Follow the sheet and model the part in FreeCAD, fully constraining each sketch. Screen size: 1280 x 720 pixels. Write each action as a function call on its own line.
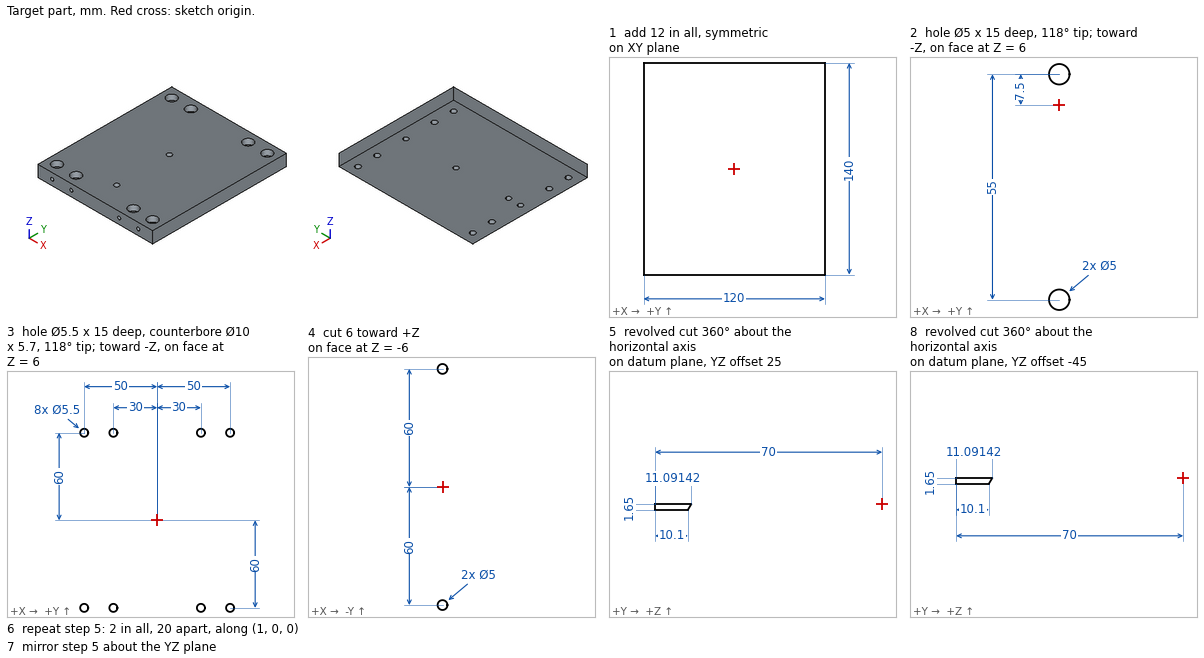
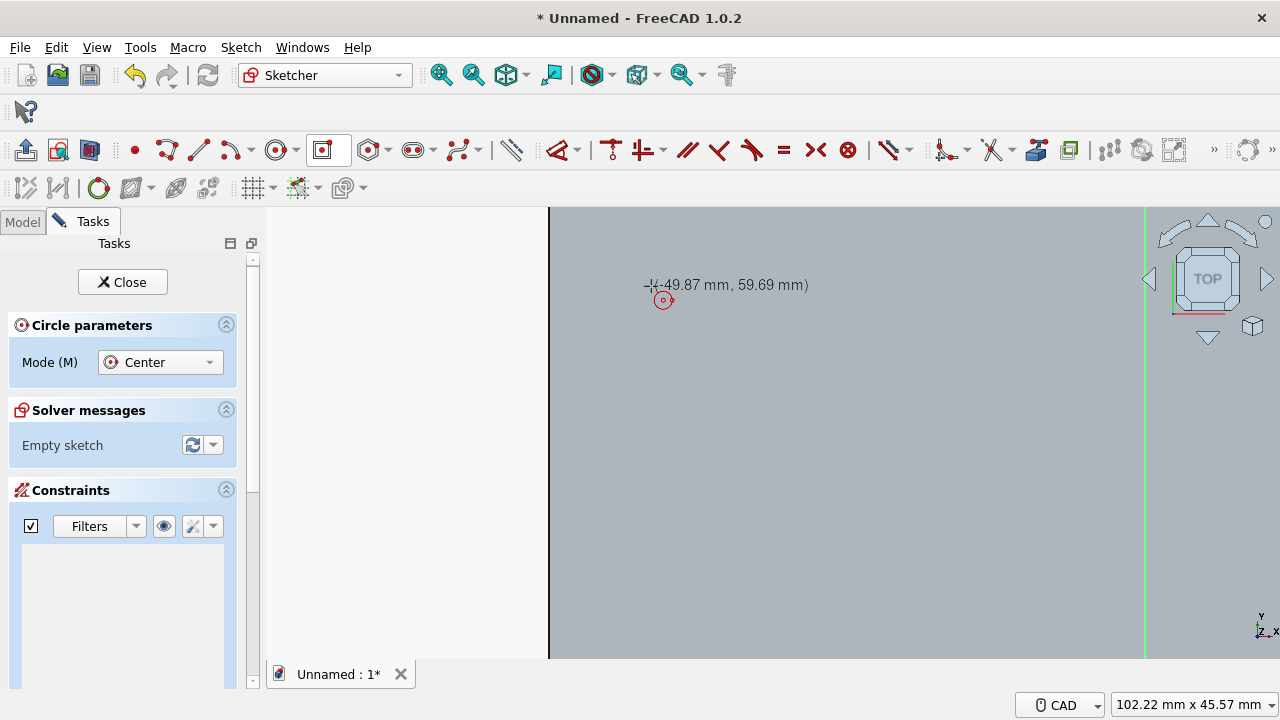
scroll(560, 286, down, 7)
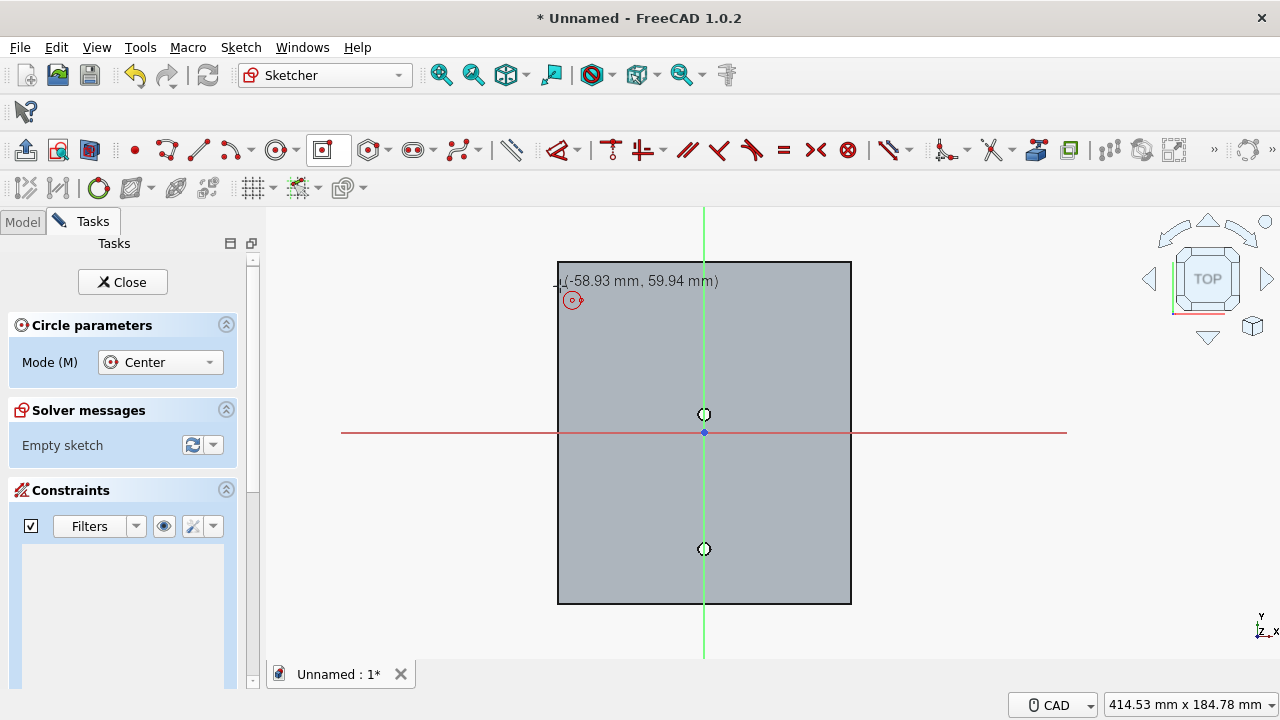
click(582, 286)
move(587, 281)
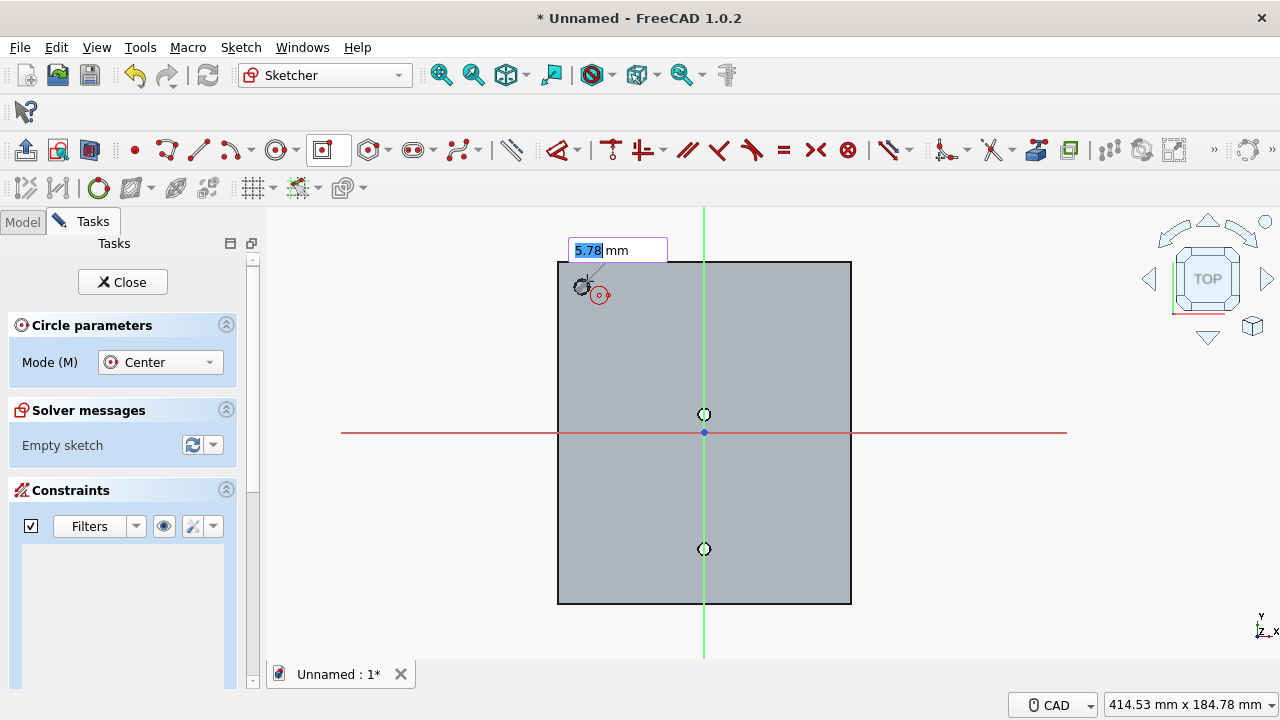
text(5.5)
key(Return)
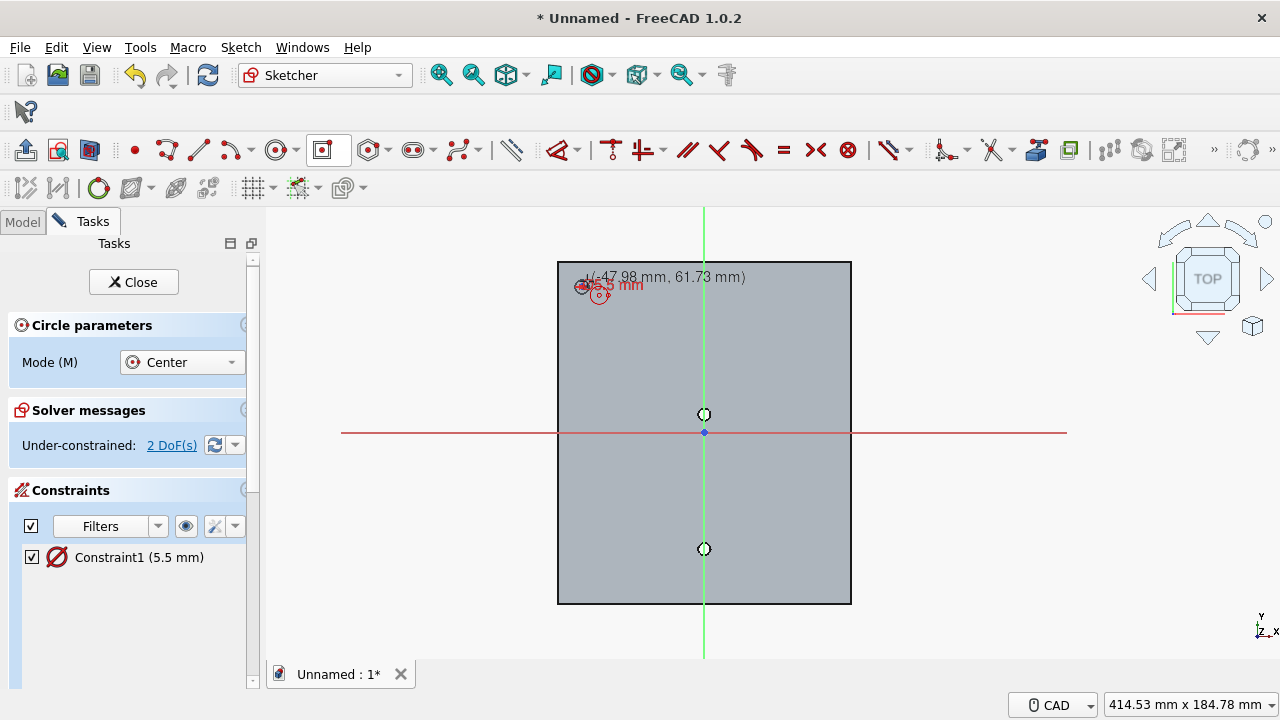
scroll(631, 286, up, 7)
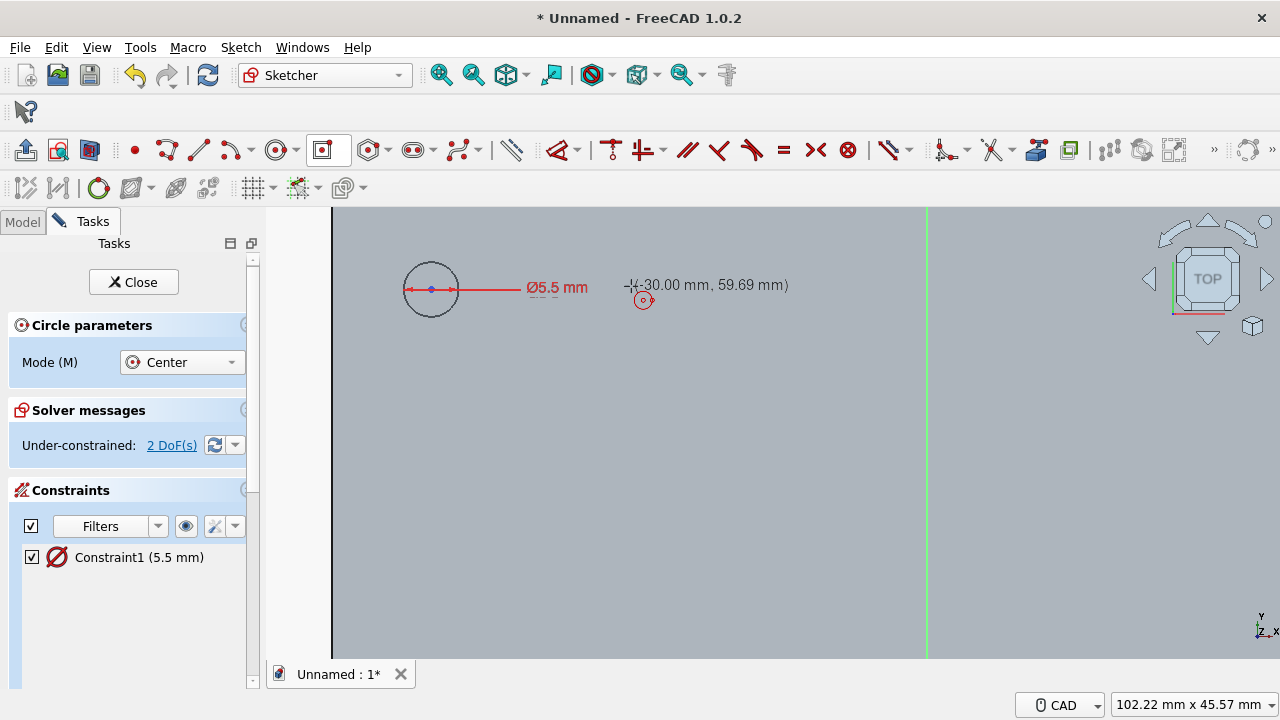
scroll(632, 286, down, 7)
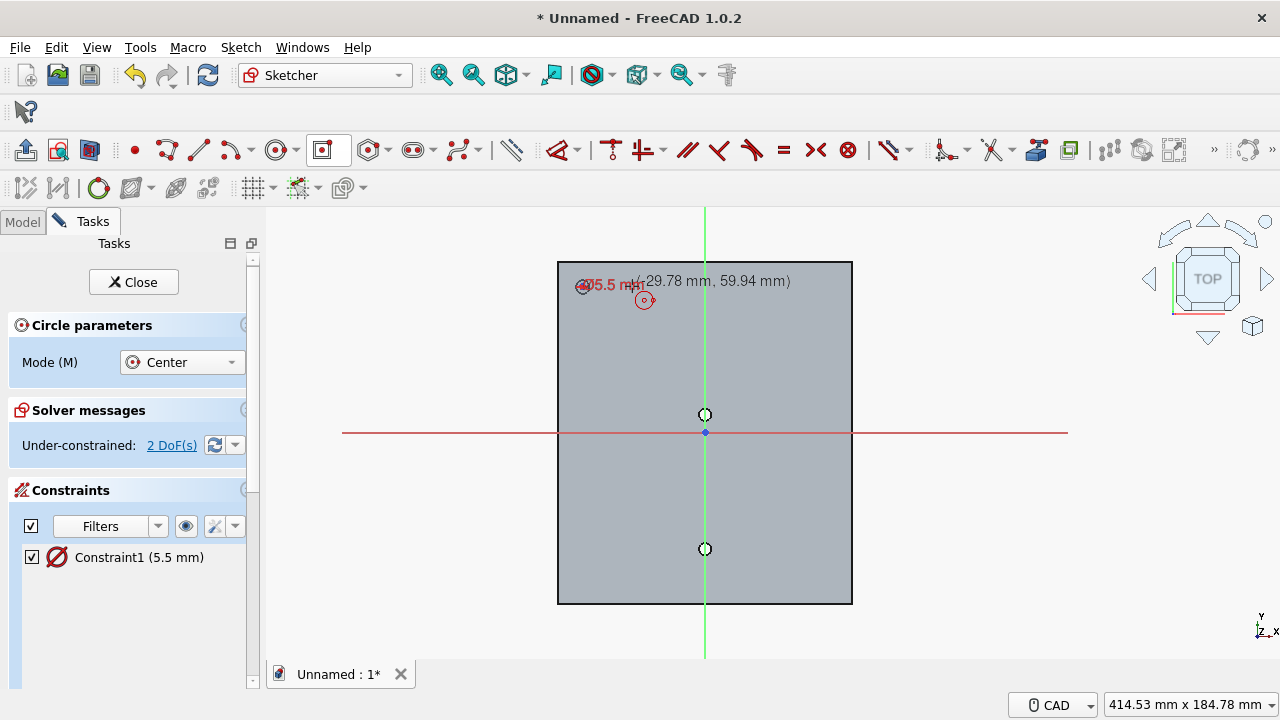
click(632, 286)
move(636, 281)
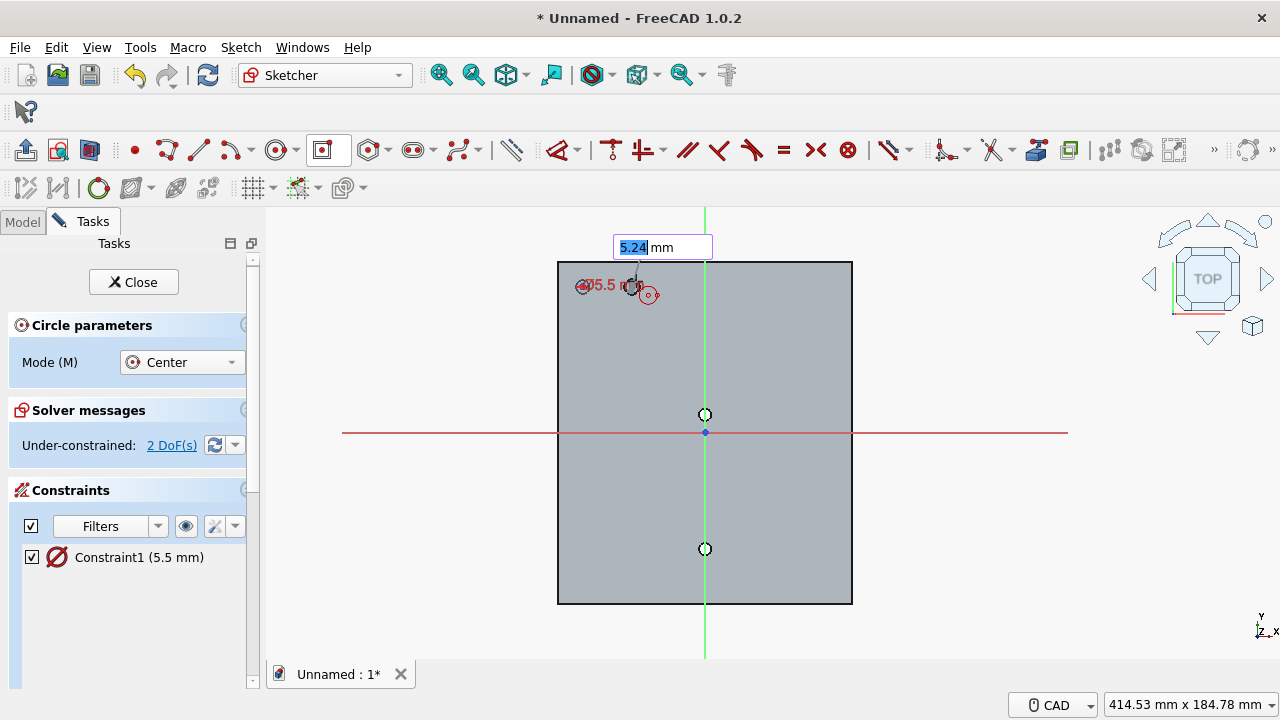
text(5.5)
key(Return)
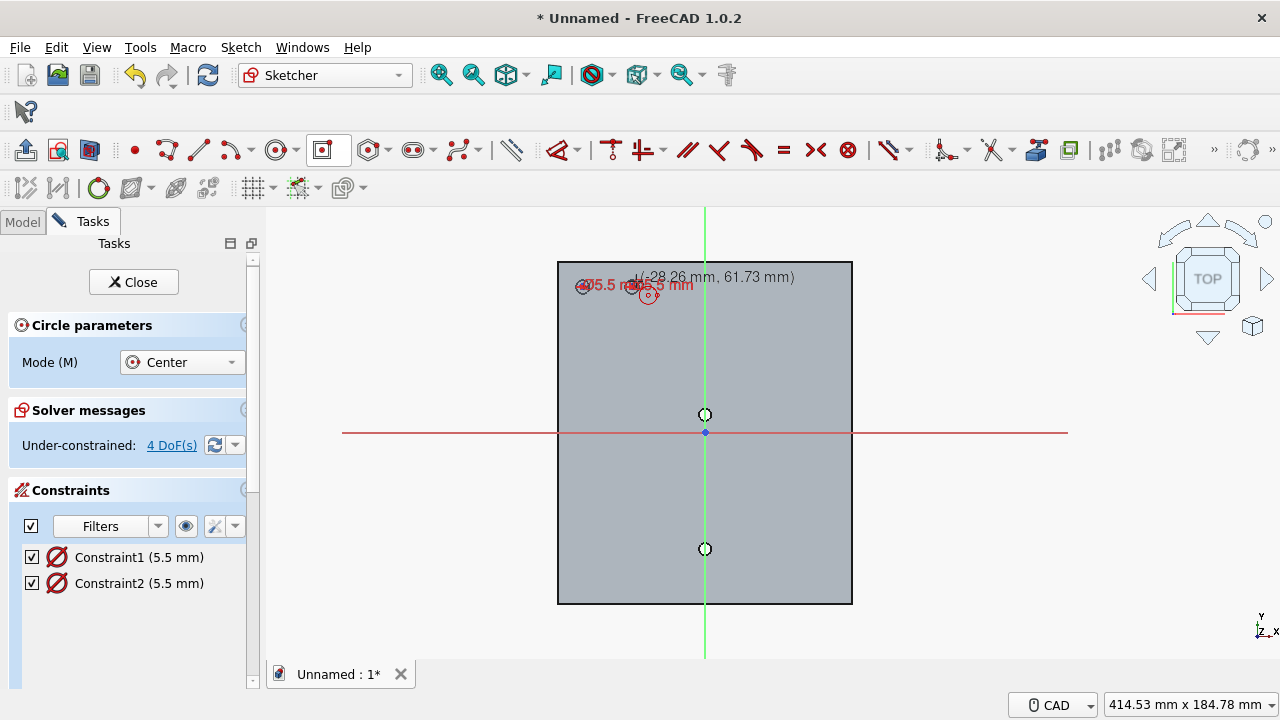
scroll(779, 286, up, 7)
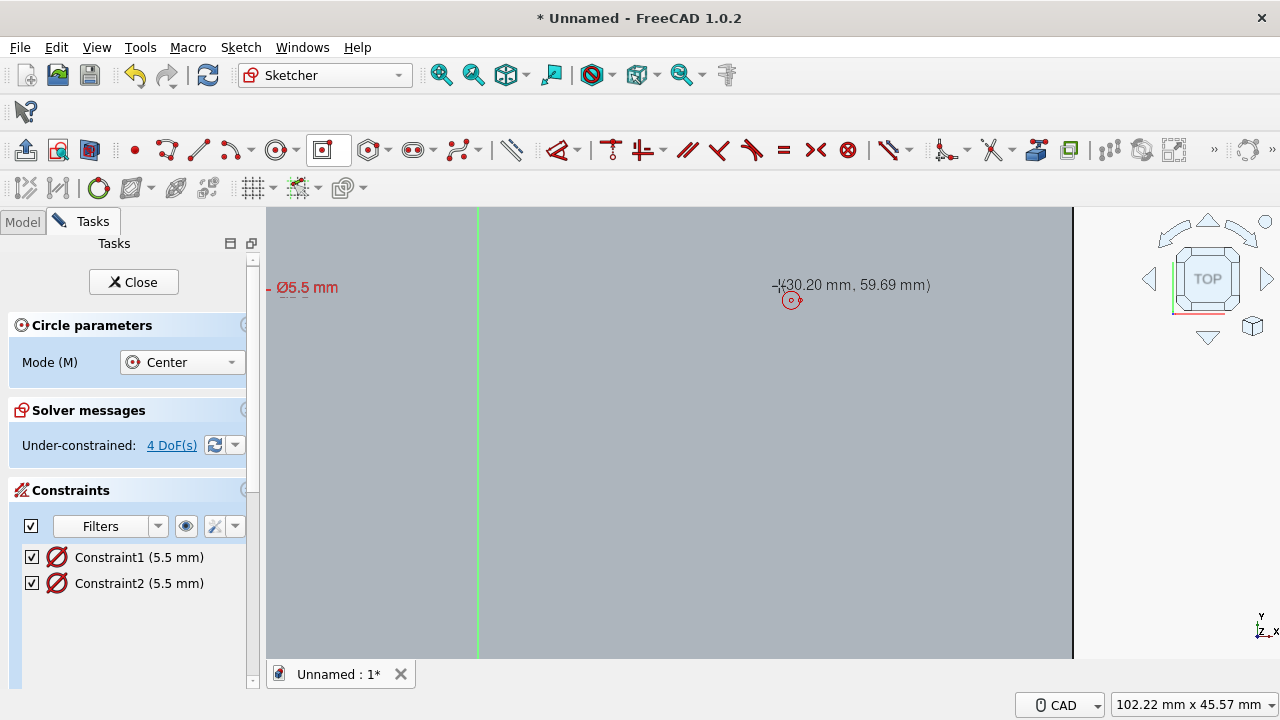
scroll(779, 286, down, 7)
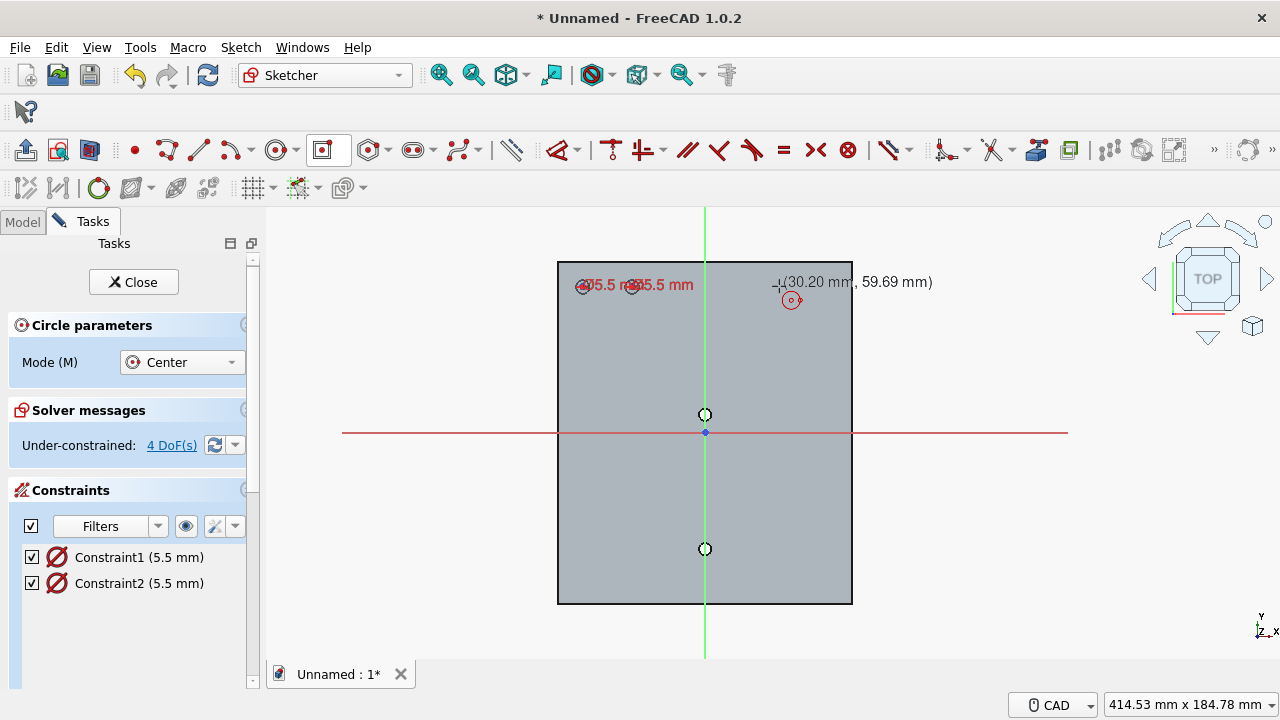
click(779, 286)
move(783, 281)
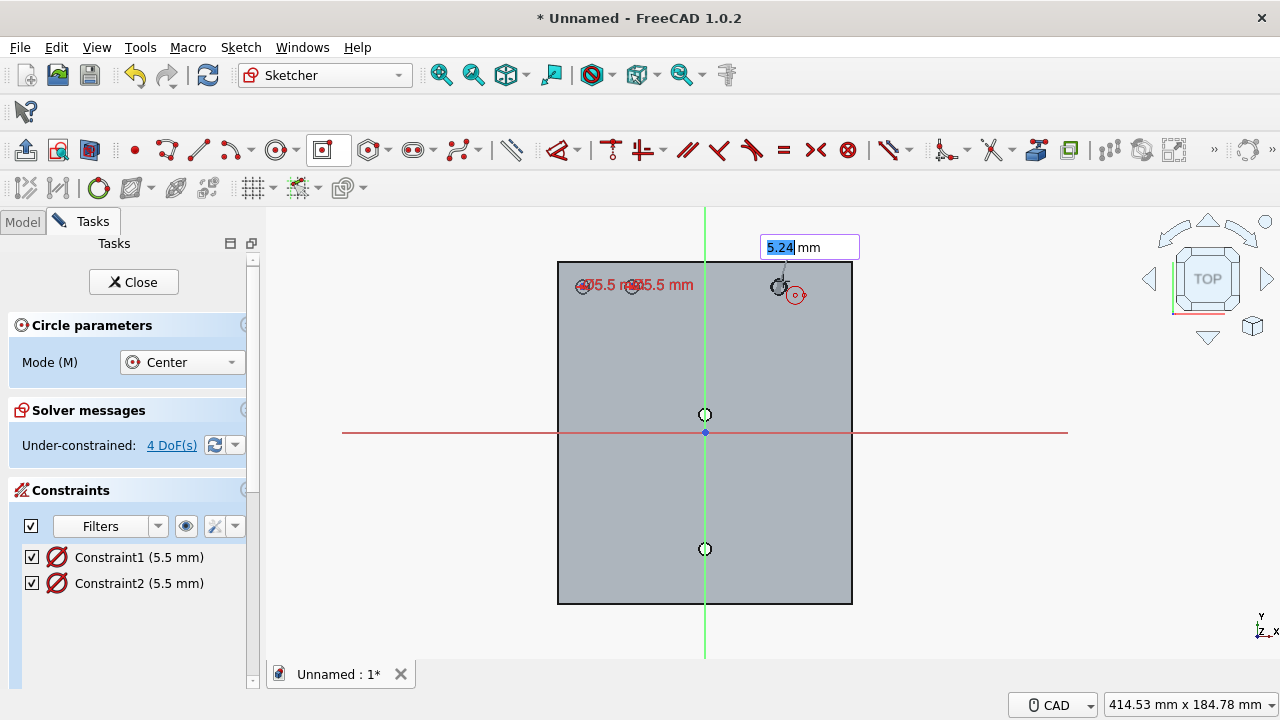
text(5.5)
key(Return)